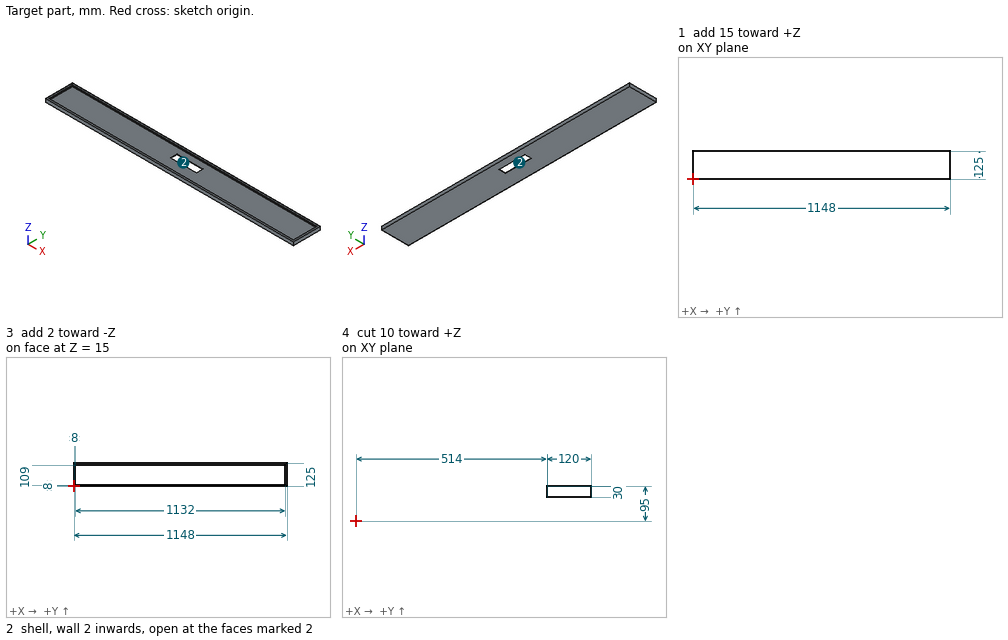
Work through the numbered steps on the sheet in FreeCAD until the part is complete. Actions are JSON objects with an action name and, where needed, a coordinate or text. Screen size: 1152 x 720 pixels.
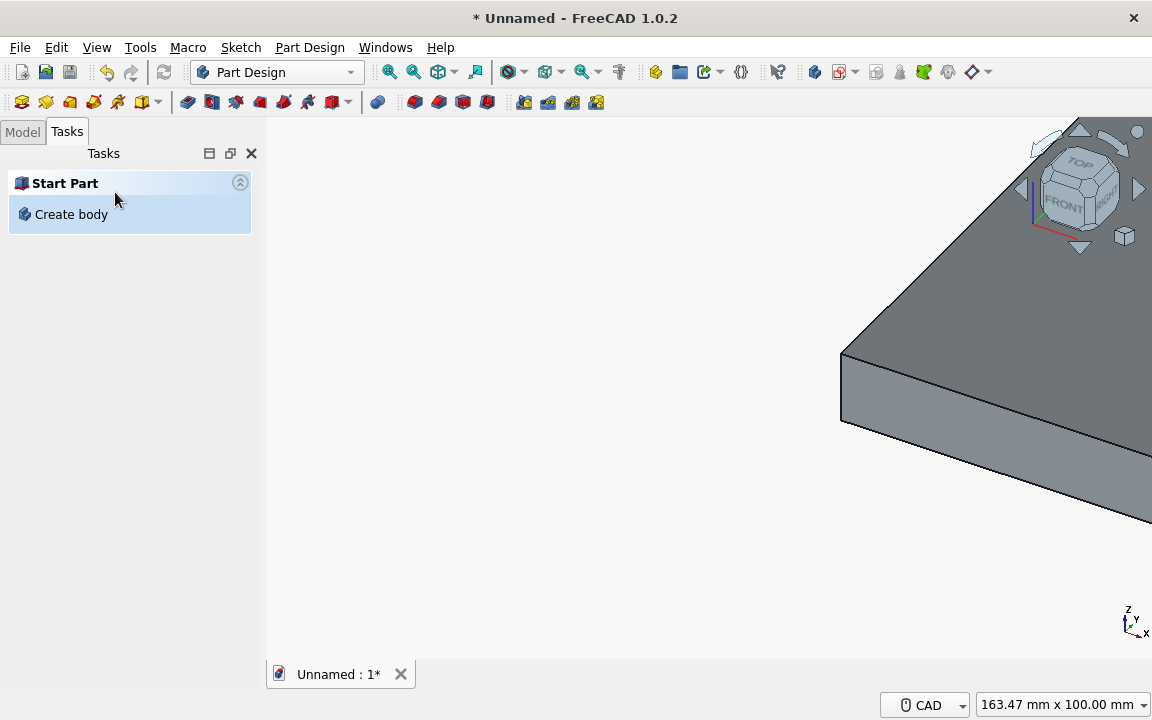
{"action": "left_click", "coordinate": [390, 72]}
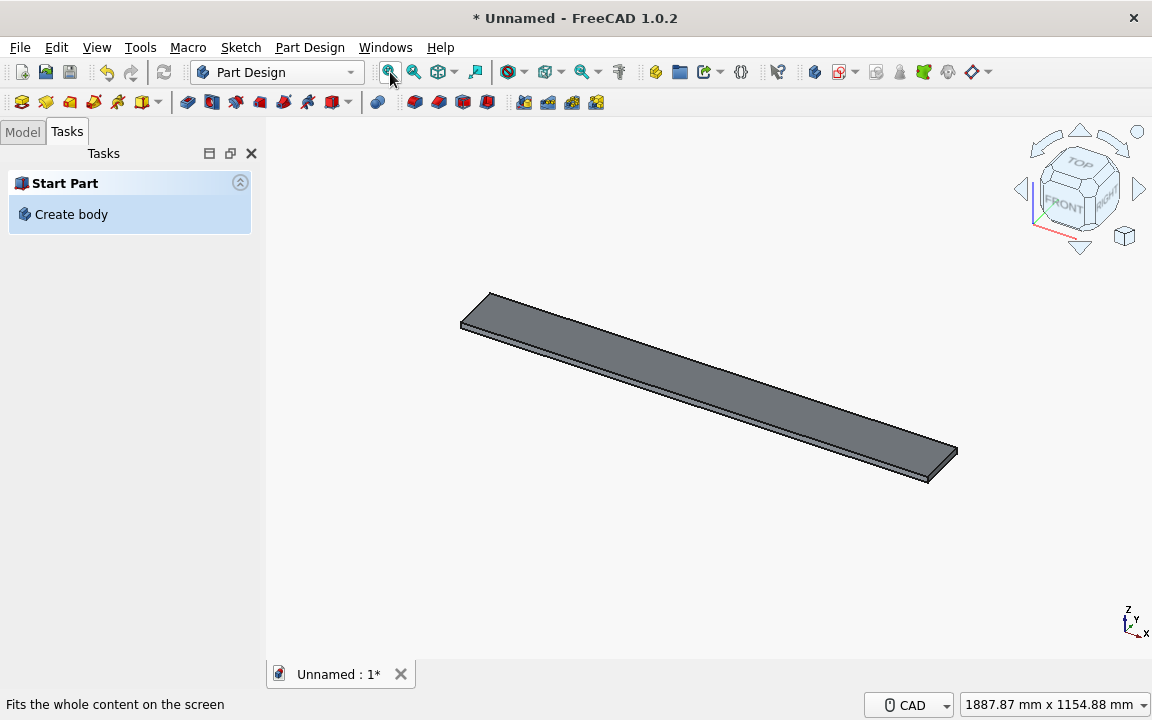
{"action": "left_click", "coordinate": [909, 450]}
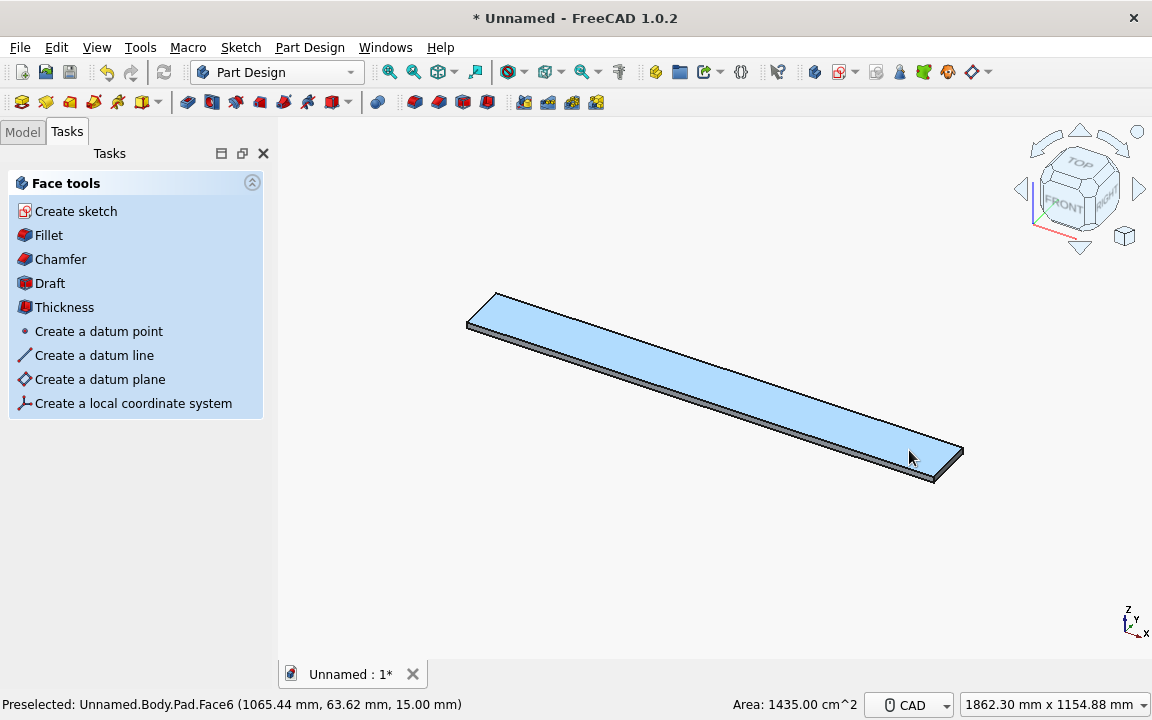
{"action": "left_click", "coordinate": [488, 102]}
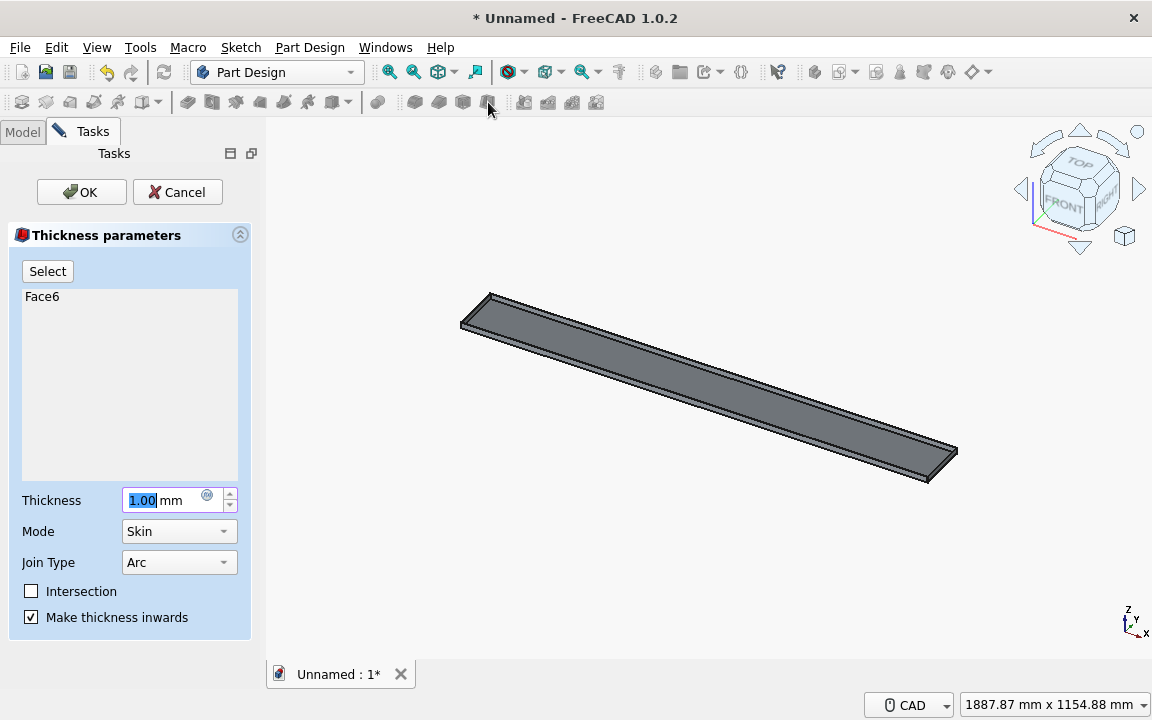
{"action": "type", "text": "2"}
{"action": "key", "text": "Tab"}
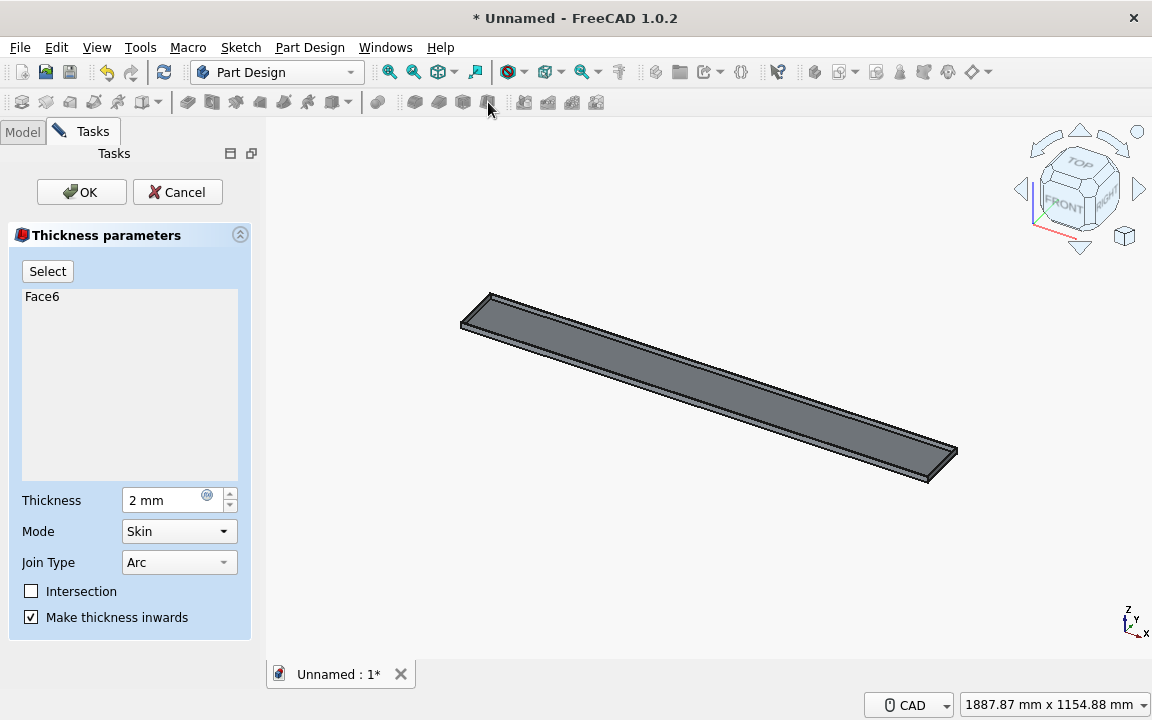
{"action": "left_click", "coordinate": [180, 562]}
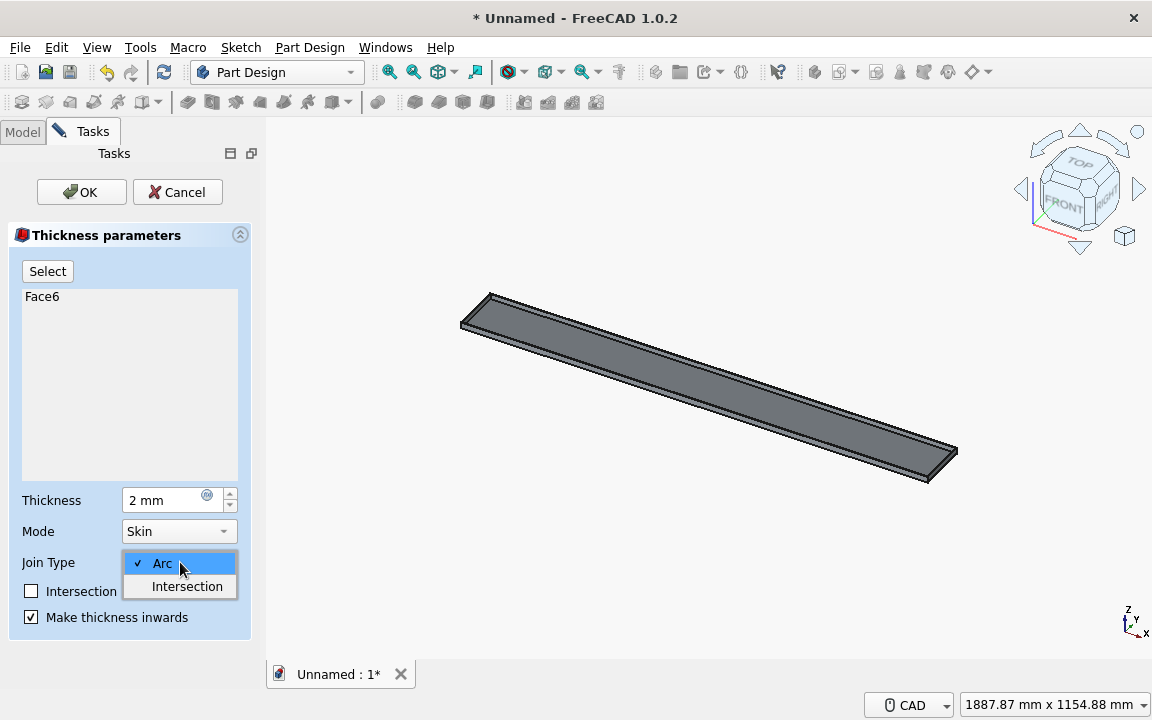
{"action": "left_click", "coordinate": [179, 586]}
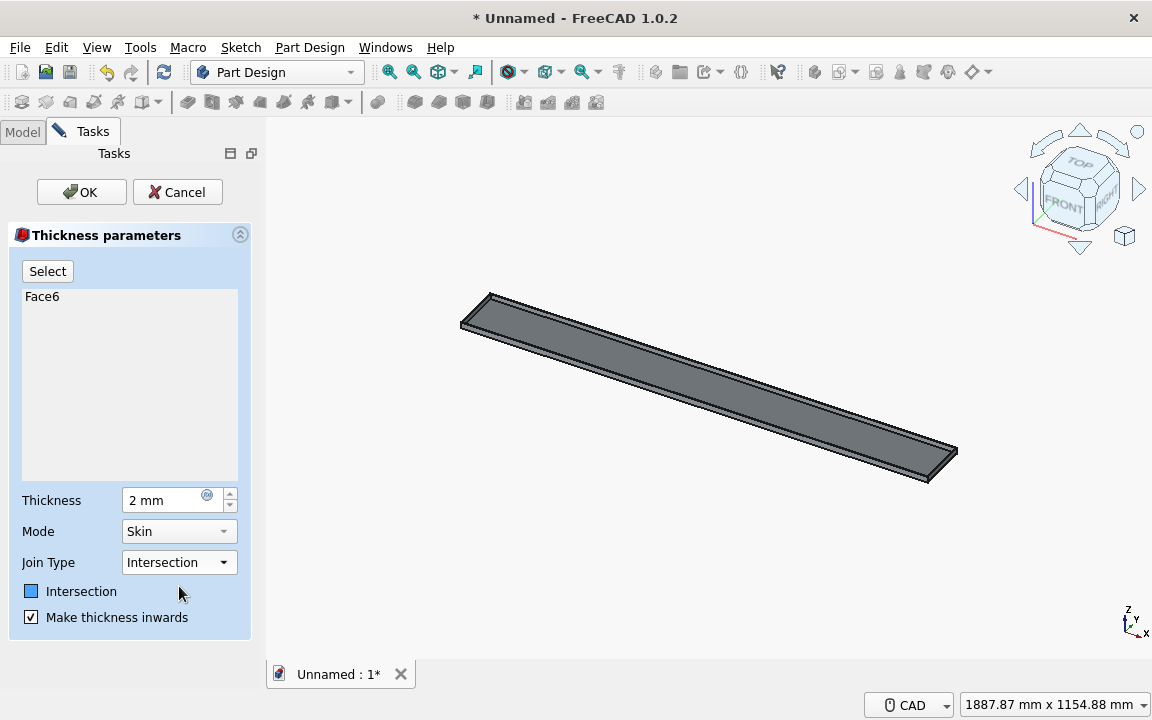
{"action": "left_click", "coordinate": [82, 192]}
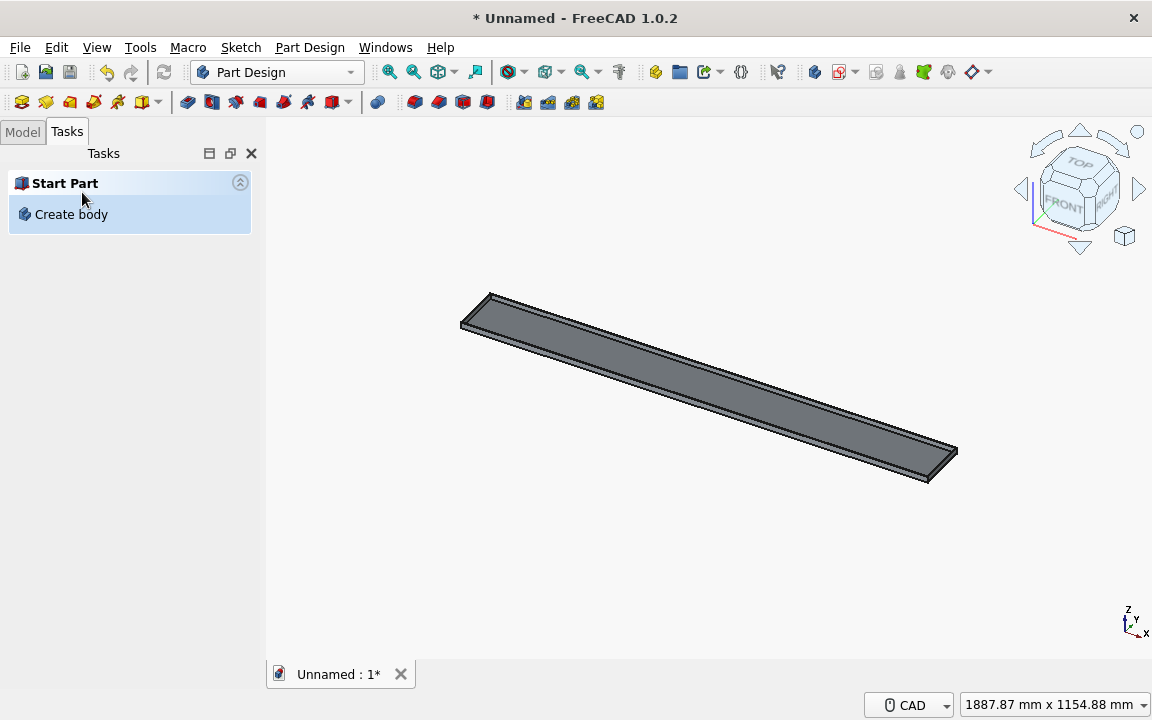
{"action": "scroll", "coordinate": [937, 466], "scroll_direction": "up", "scroll_amount": 15}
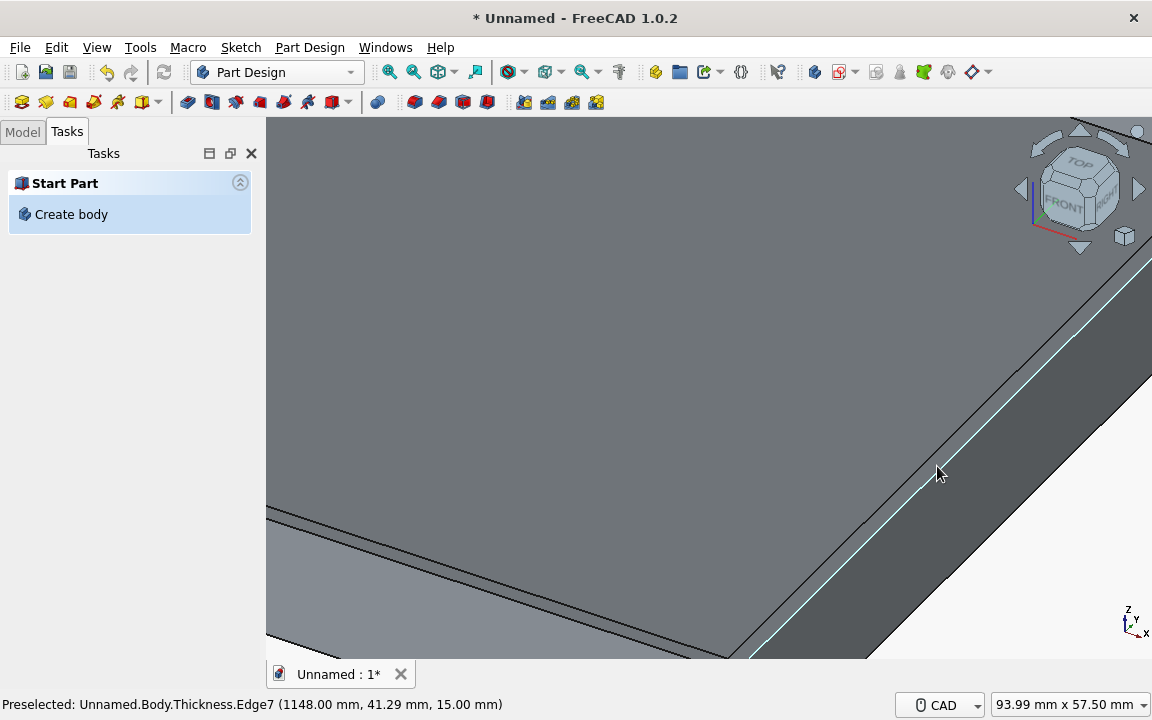
{"action": "scroll", "coordinate": [928, 472], "scroll_direction": "up", "scroll_amount": 4}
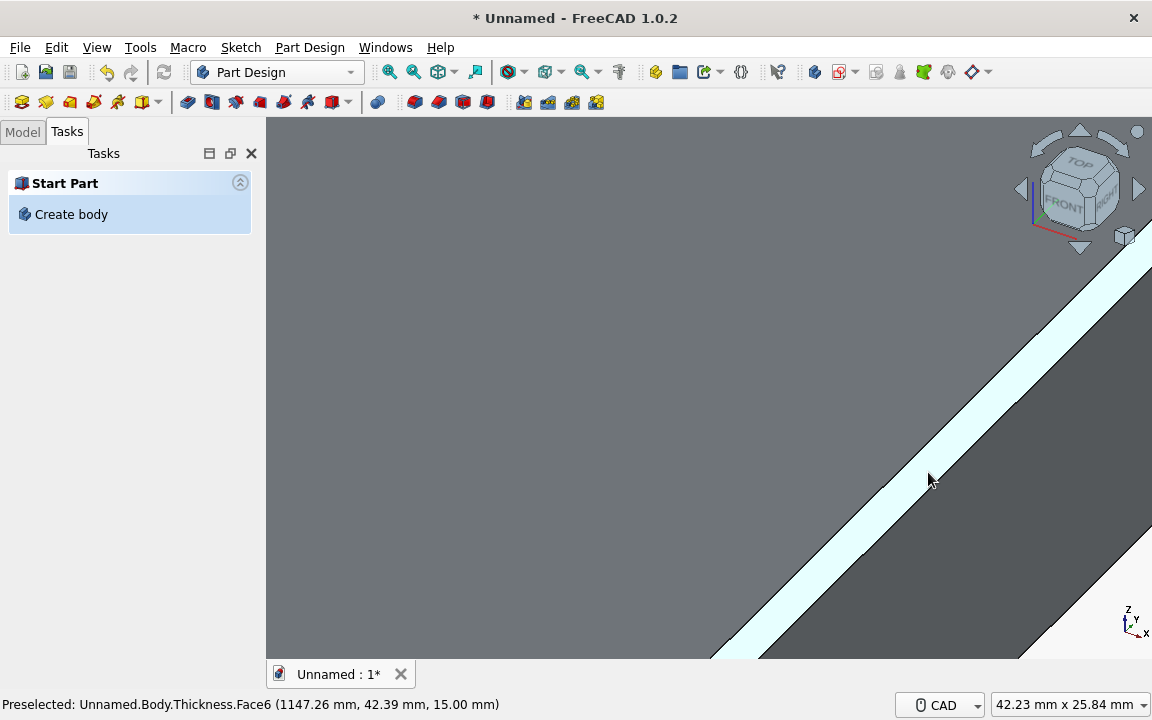
{"action": "left_click", "coordinate": [928, 473]}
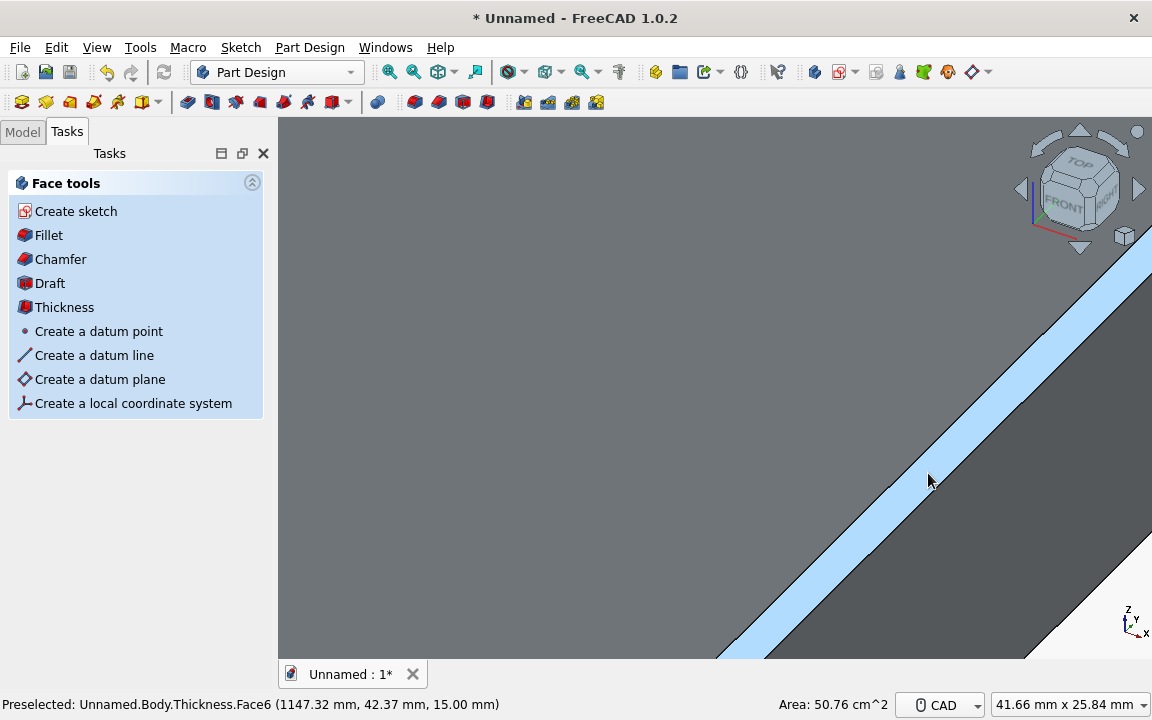
{"action": "left_click", "coordinate": [840, 72]}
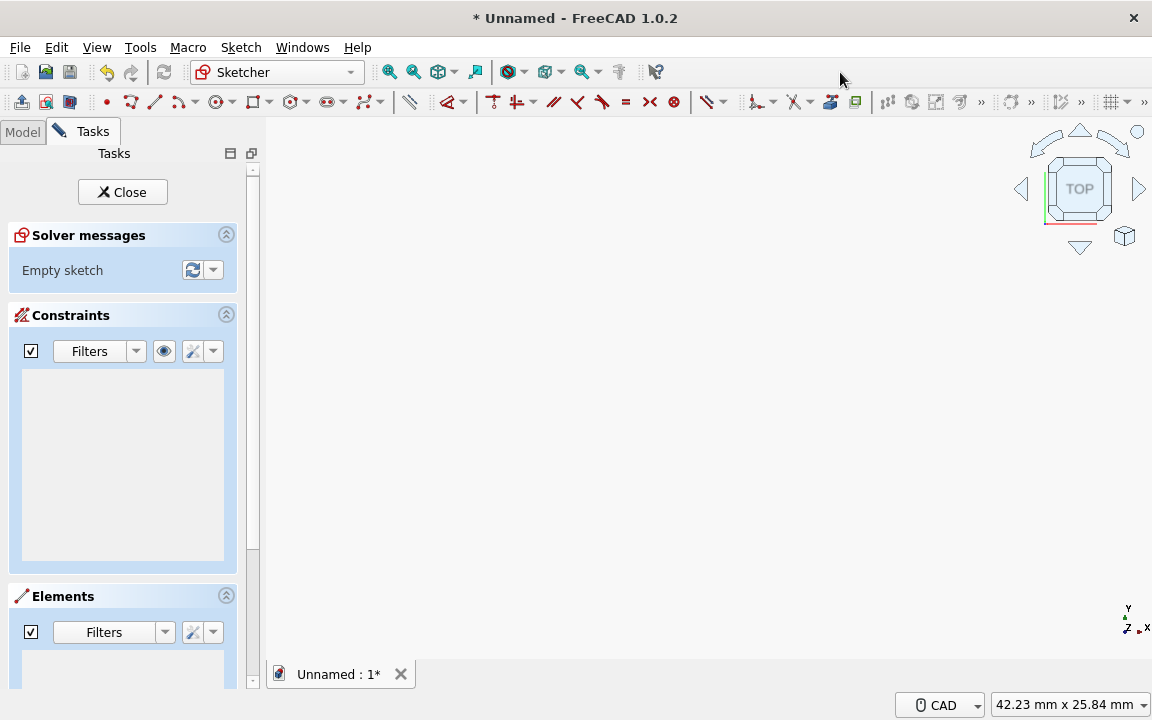
{"action": "scroll", "coordinate": [640, 388], "scroll_direction": "down", "scroll_amount": 15}